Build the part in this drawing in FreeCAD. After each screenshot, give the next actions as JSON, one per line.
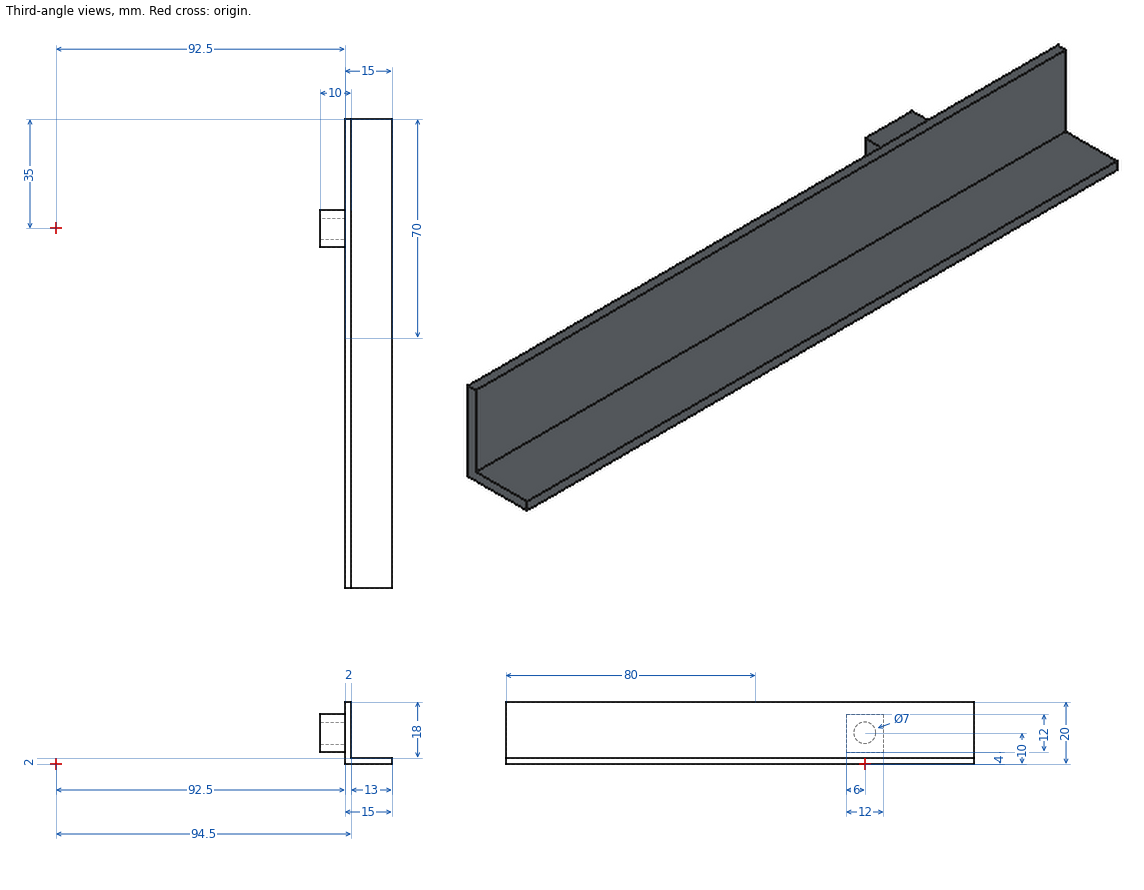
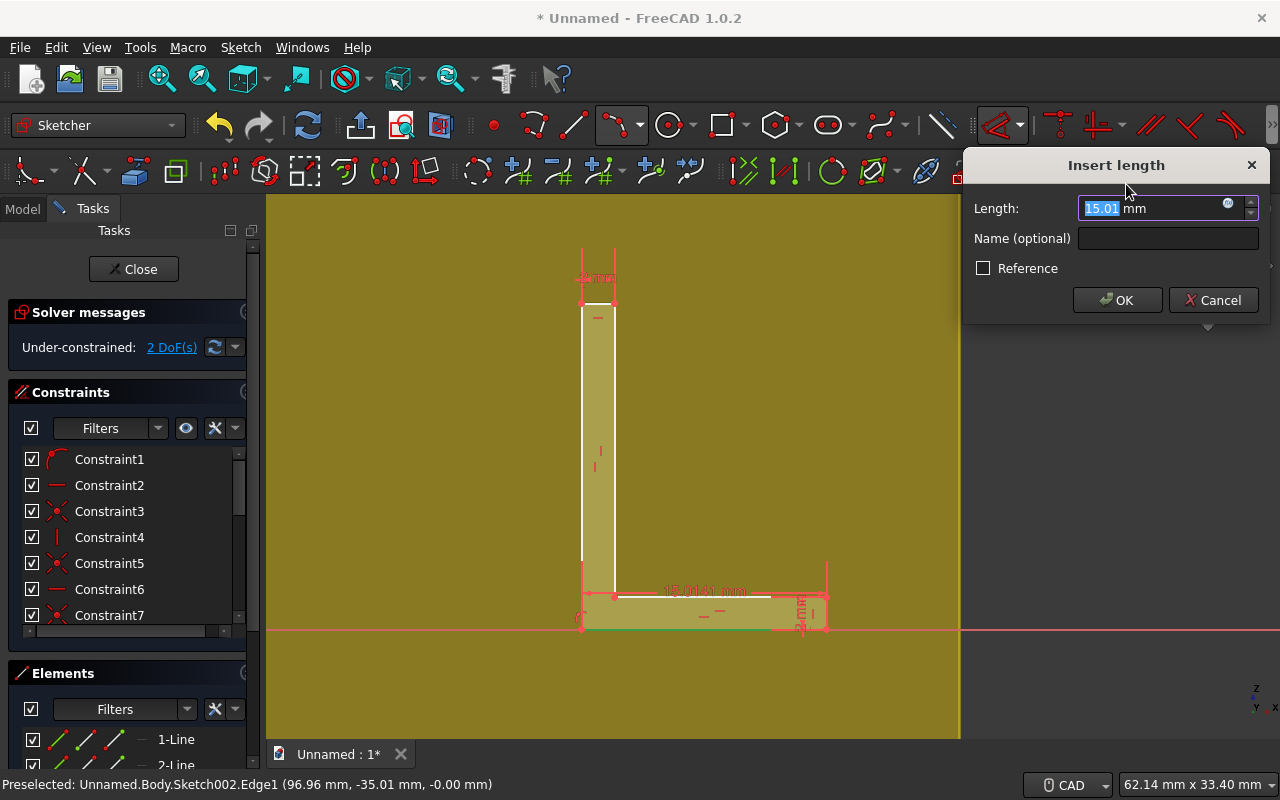
{"action": "type", "text": "15"}
{"action": "key", "text": "Return"}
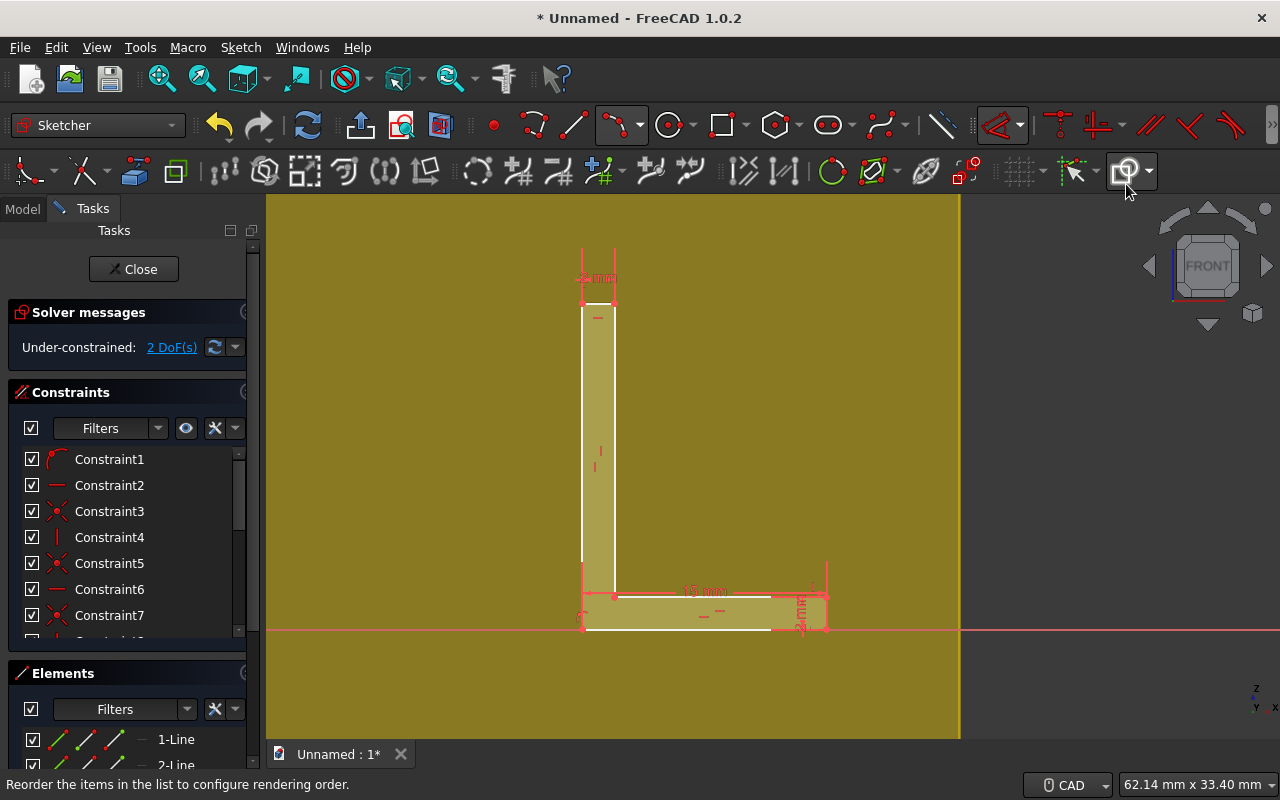
{"action": "left_click", "coordinate": [615, 509]}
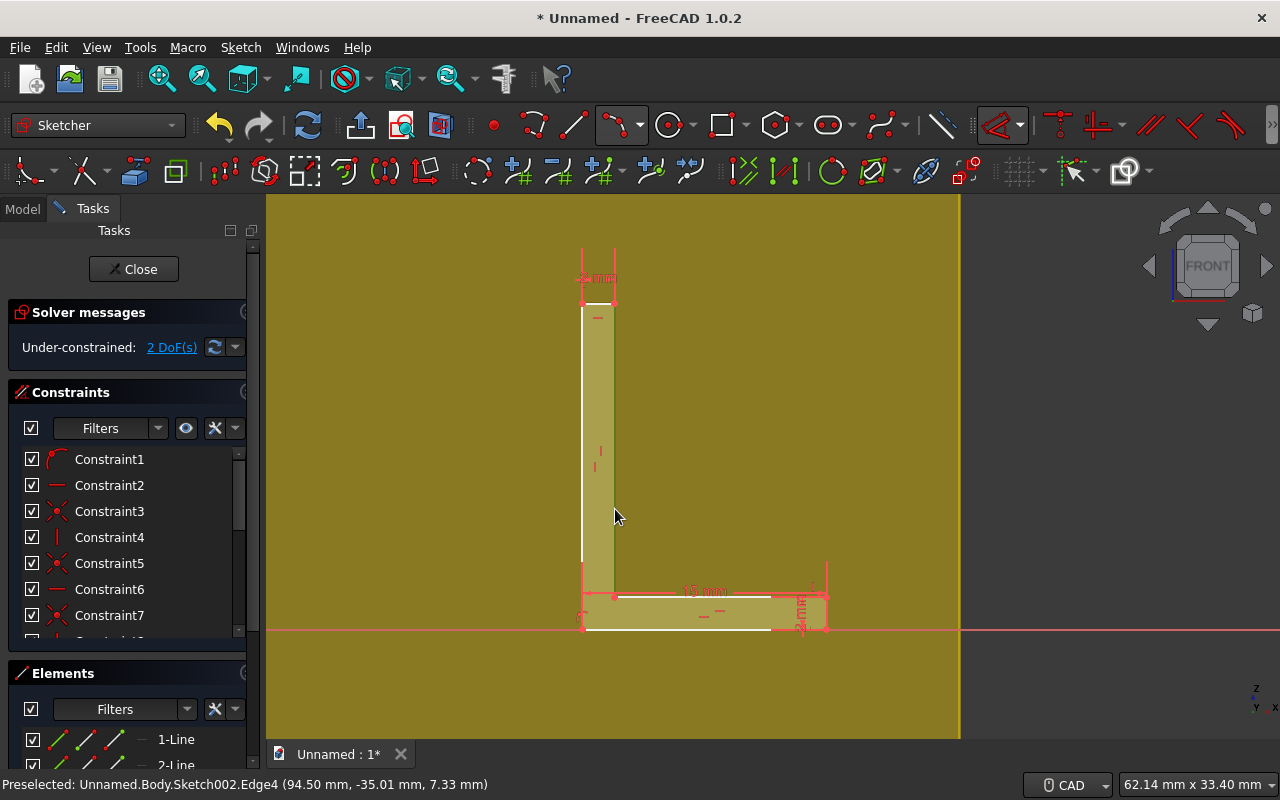
{"action": "left_click", "coordinate": [1022, 126]}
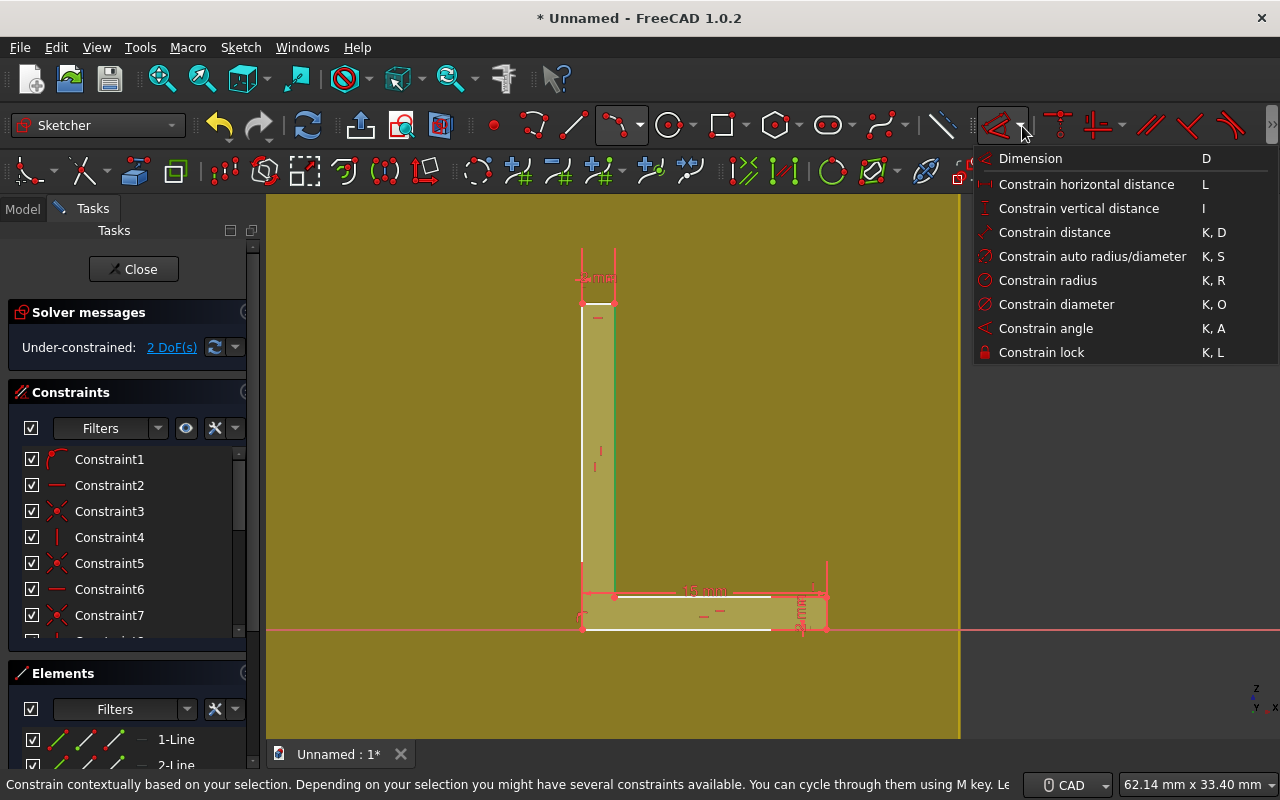
{"action": "left_click", "coordinate": [1126, 208]}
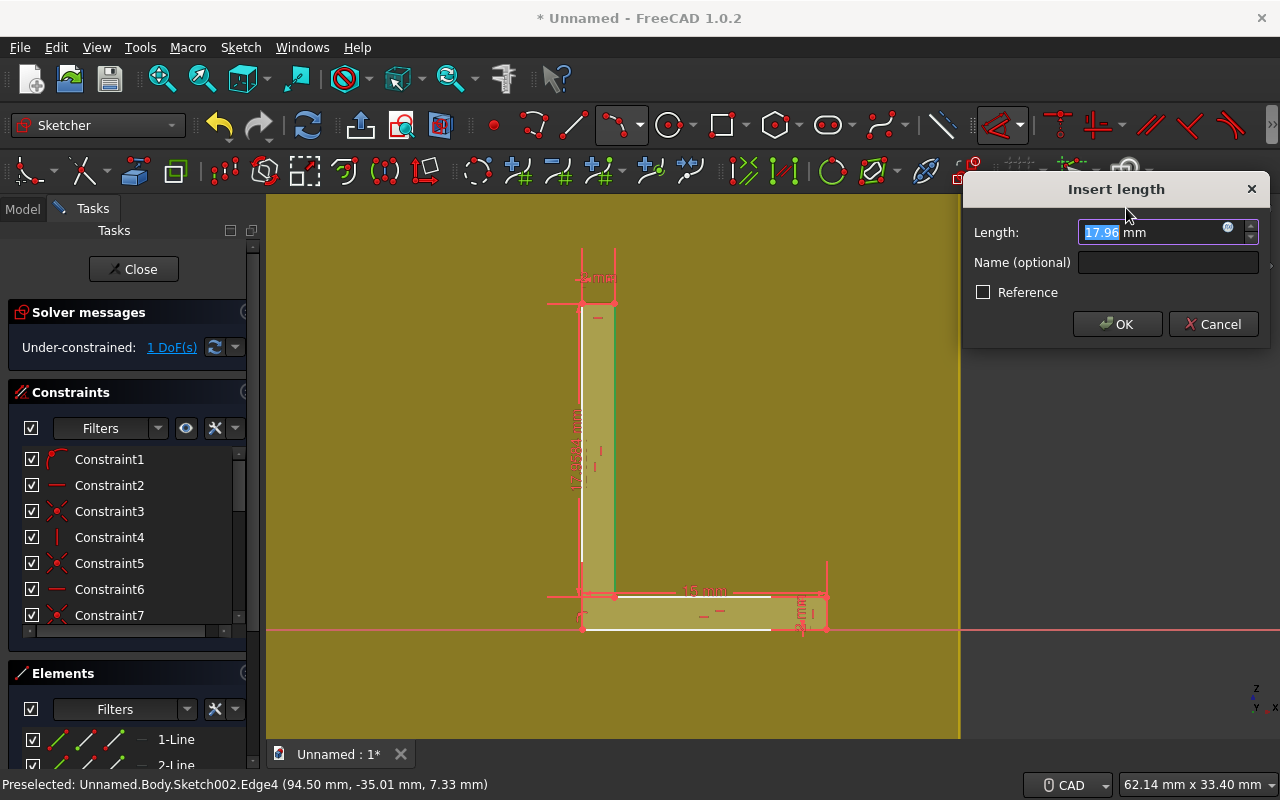
{"action": "type", "text": "18"}
{"action": "key", "text": "Return"}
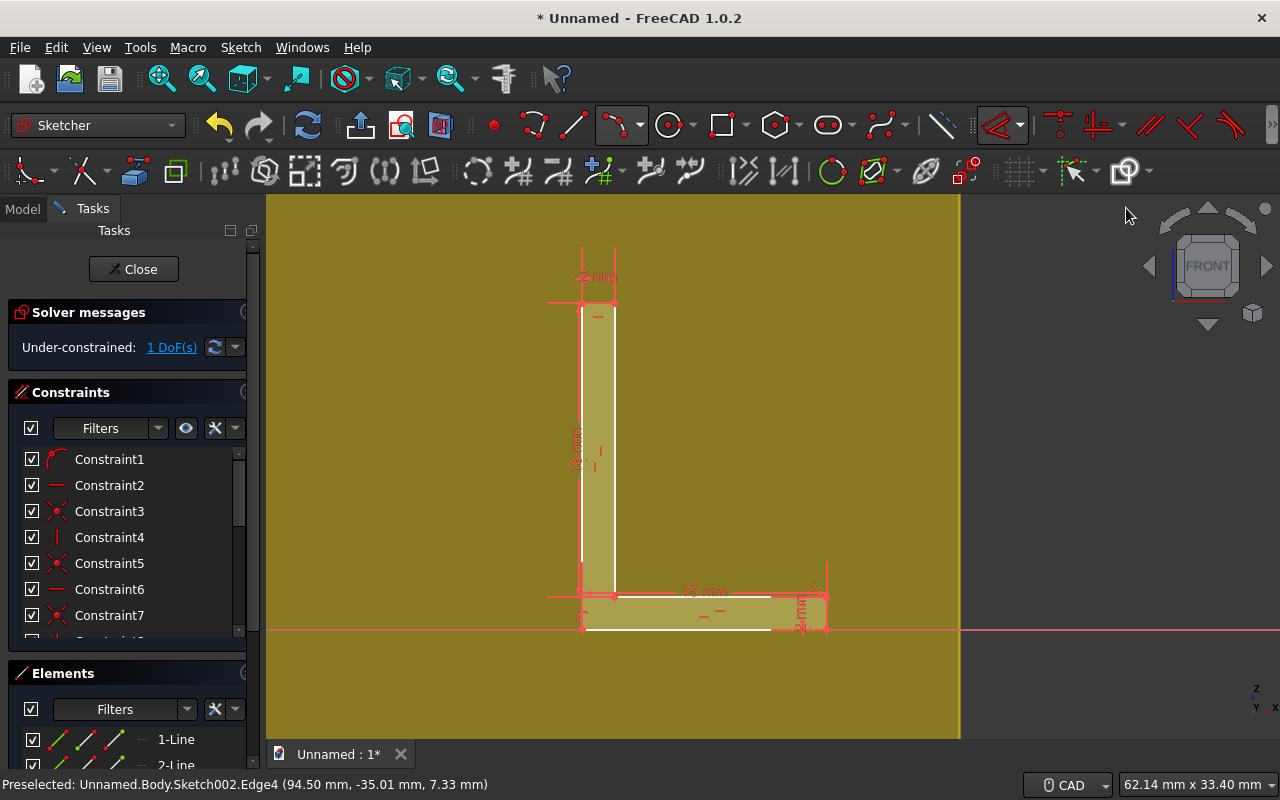
{"action": "left_click", "coordinate": [582, 630]}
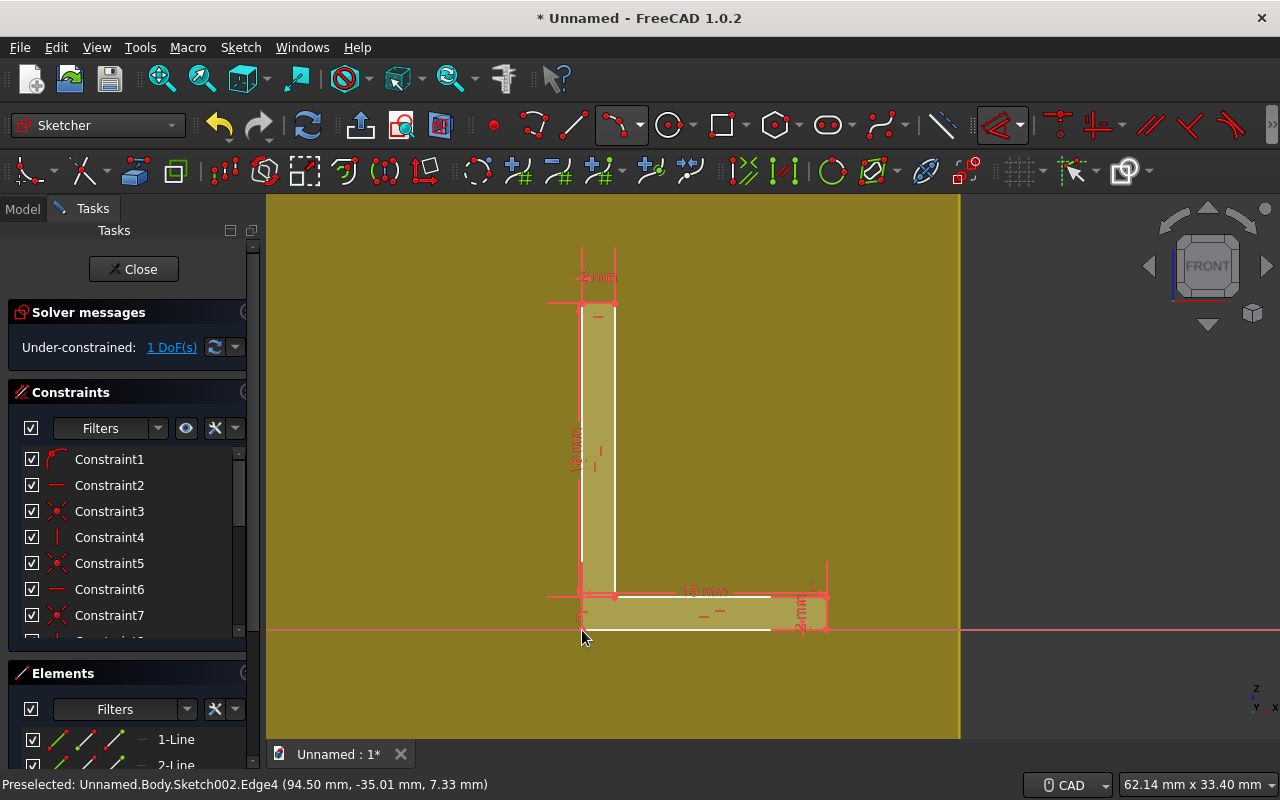
{"action": "key", "text": "l"}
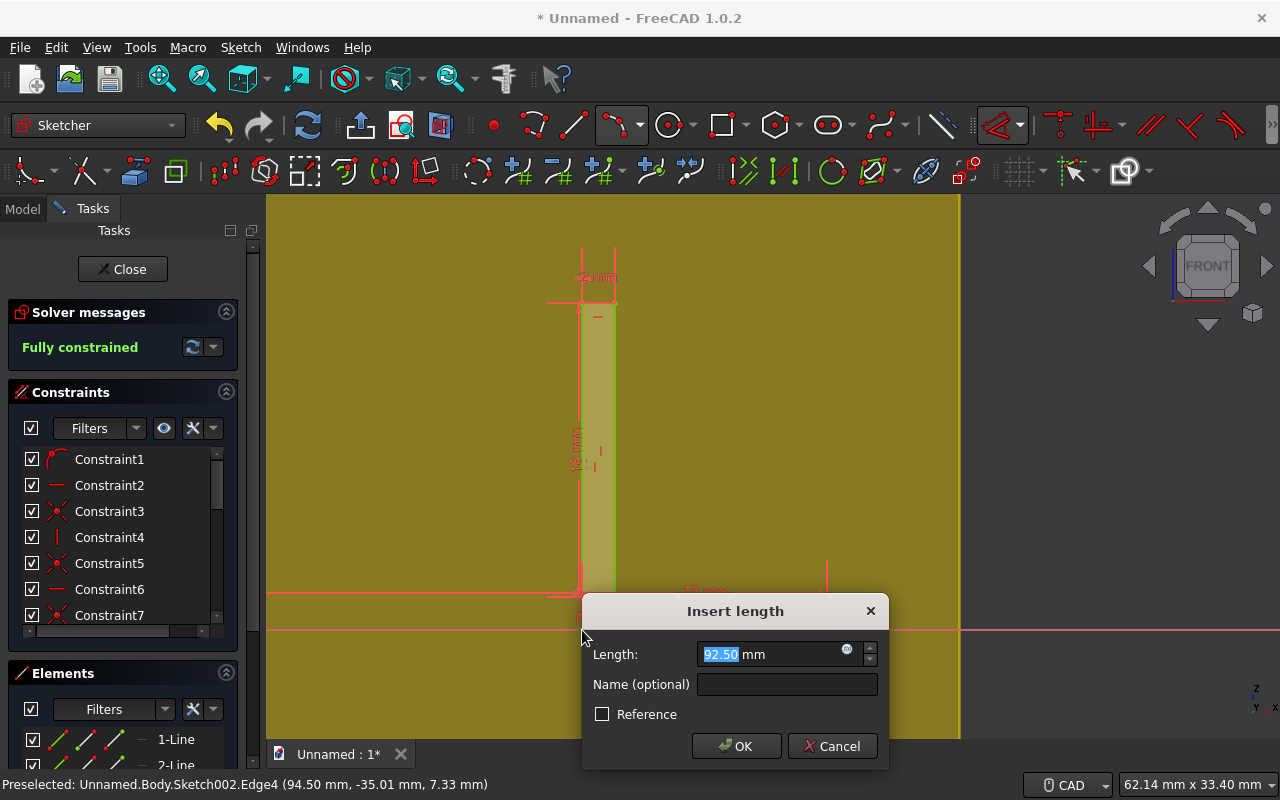
{"action": "type", "text": "92.5"}
{"action": "key", "text": "Return"}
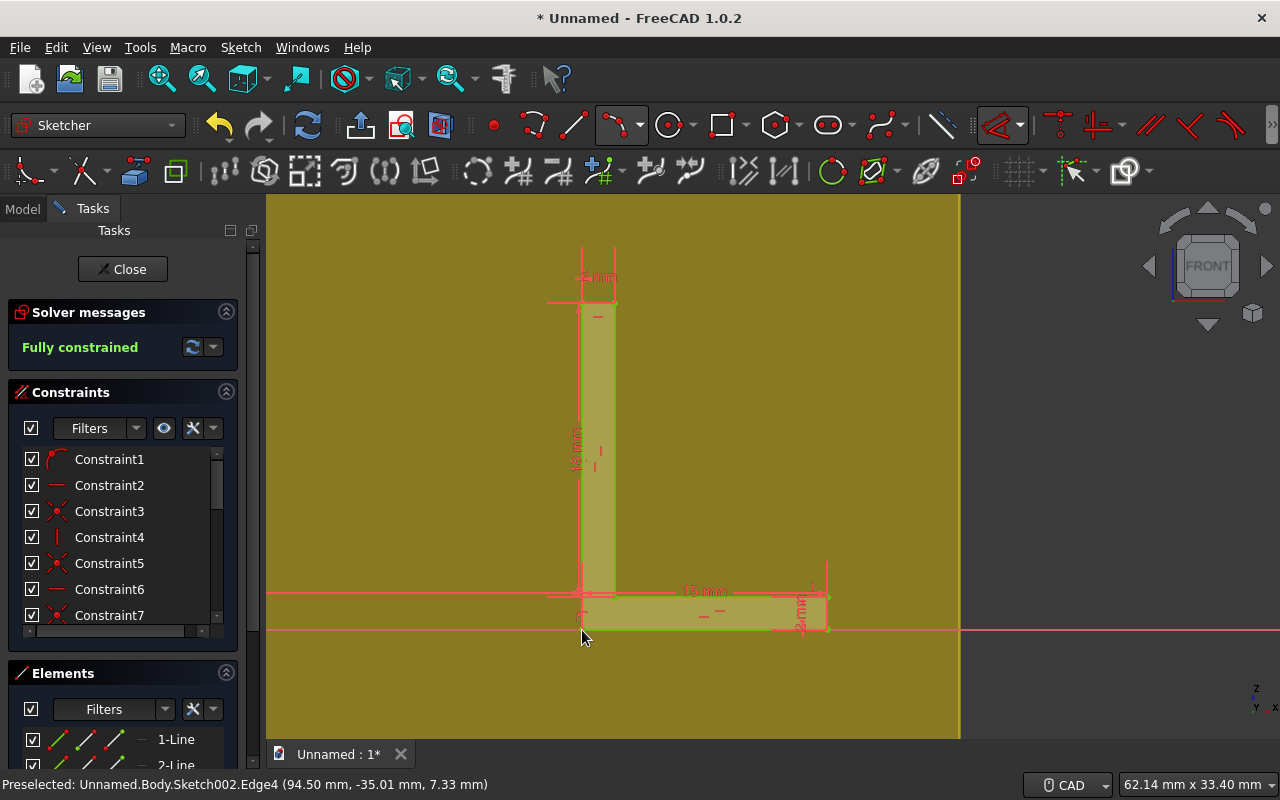
{"action": "left_click", "coordinate": [123, 269]}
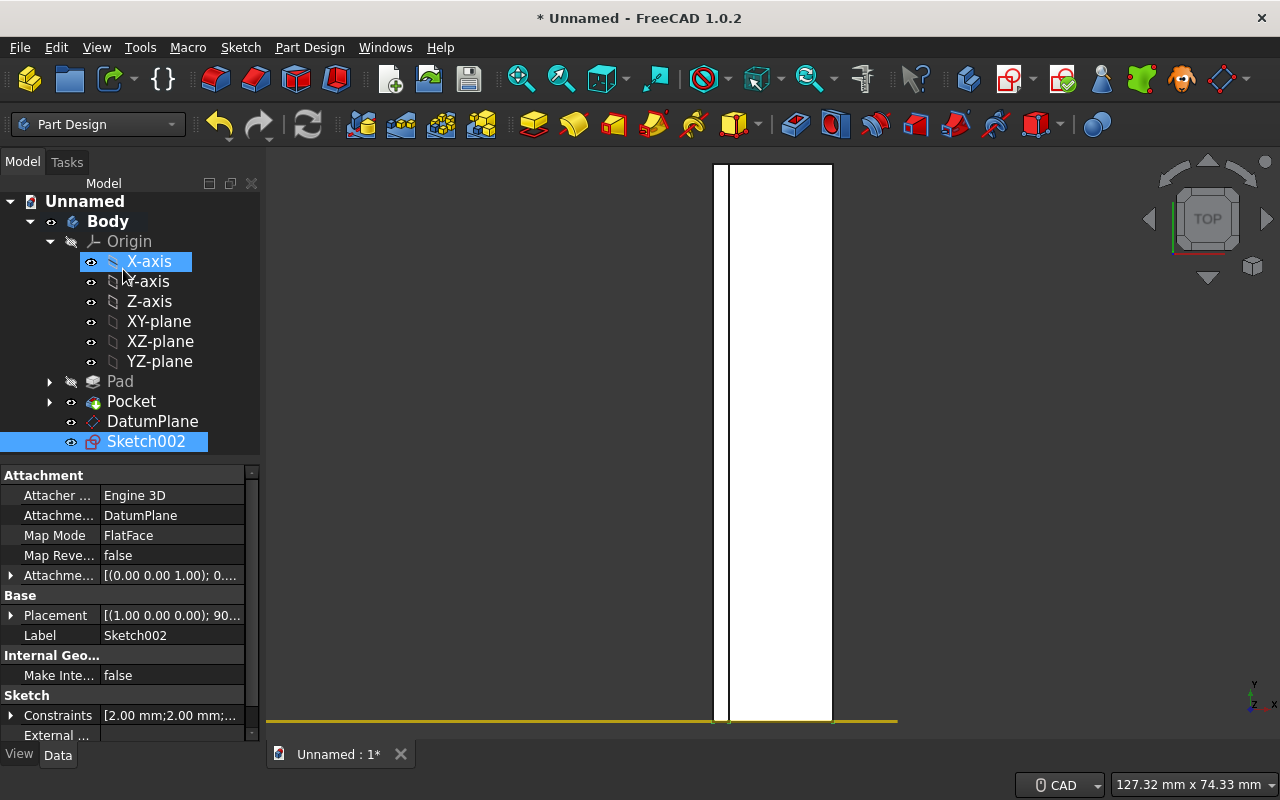
{"action": "left_click", "coordinate": [534, 124]}